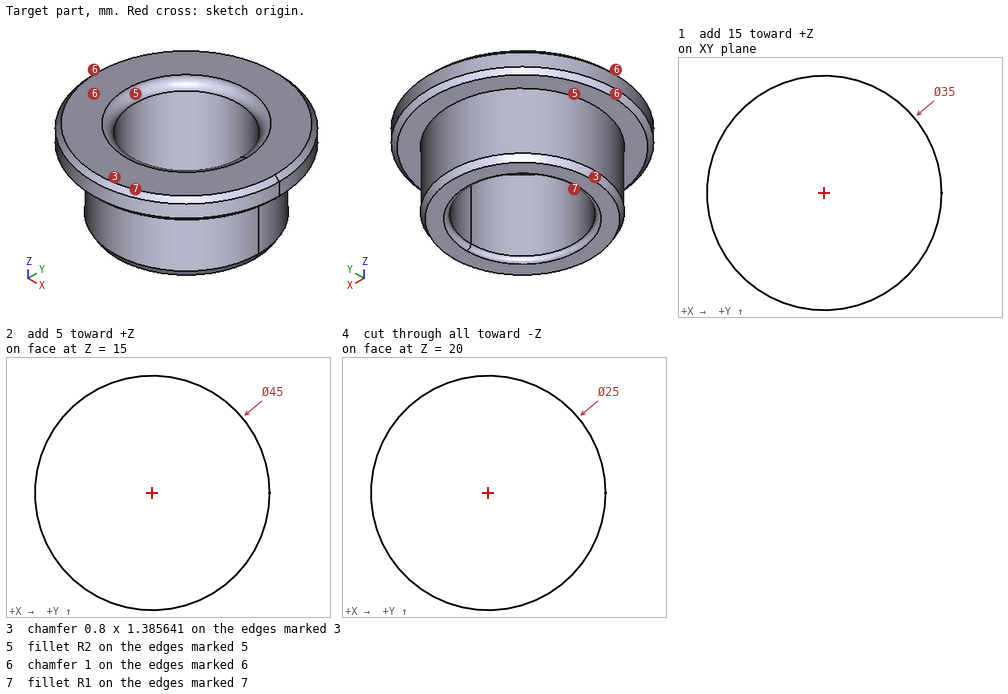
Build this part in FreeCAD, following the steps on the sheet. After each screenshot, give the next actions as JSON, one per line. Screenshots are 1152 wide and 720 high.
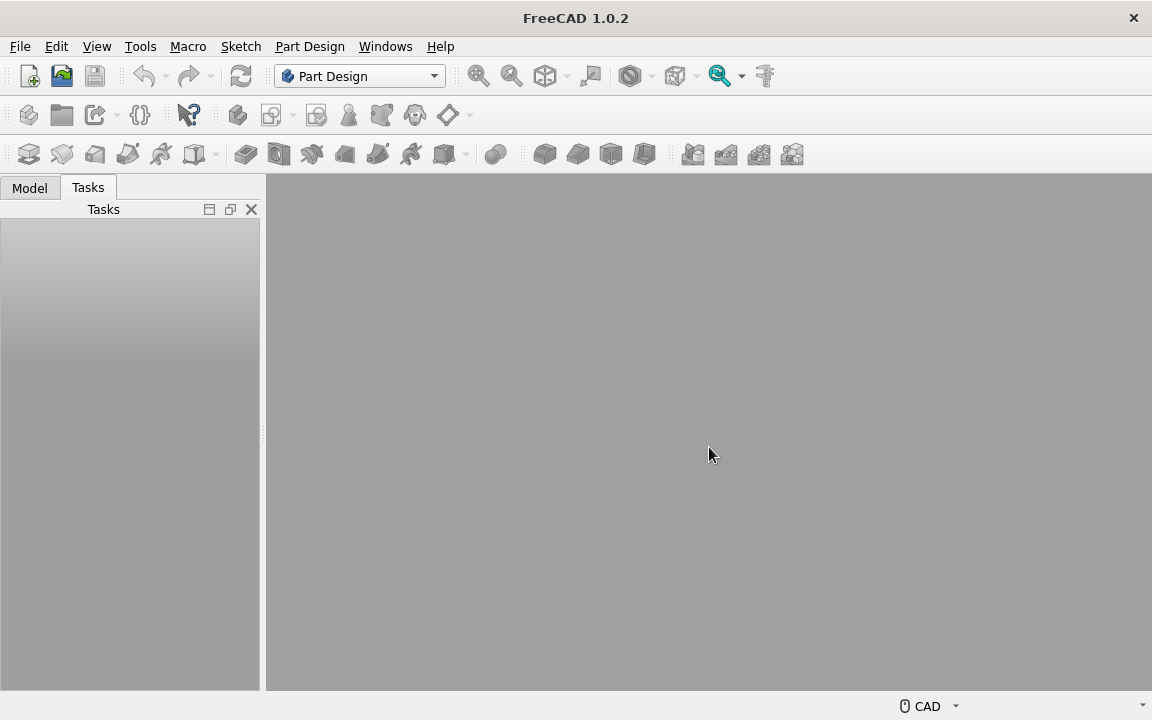
{"action": "left_click", "coordinate": [29, 76]}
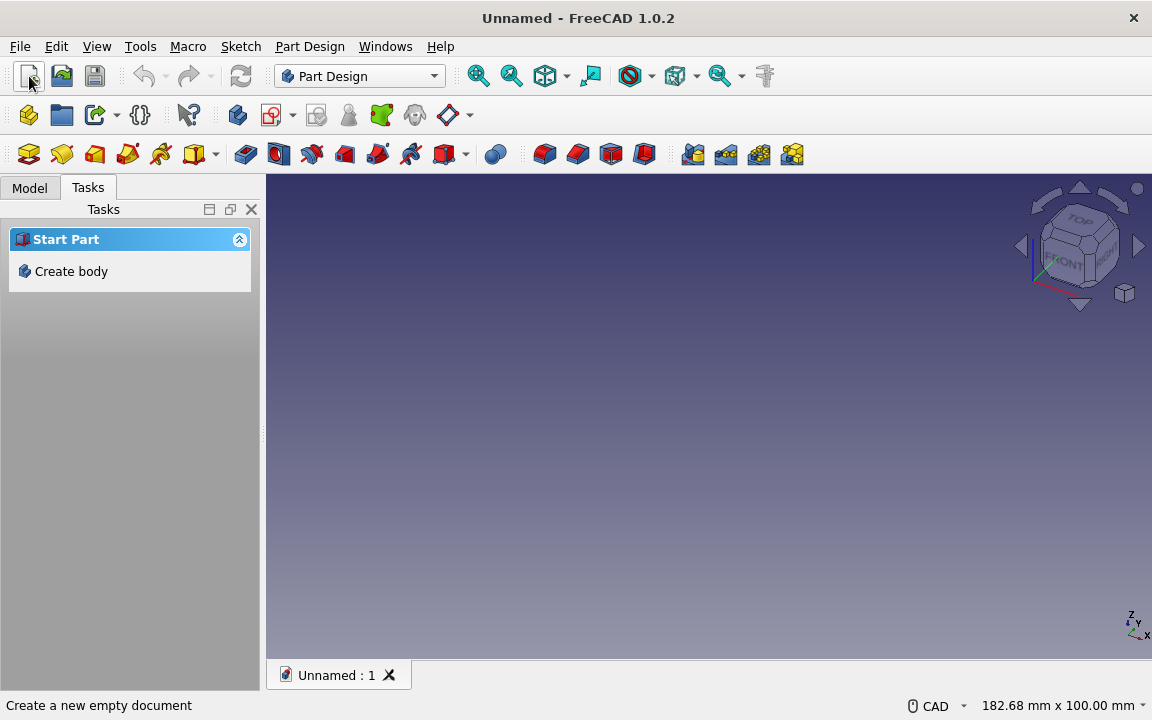
{"action": "left_click", "coordinate": [270, 116]}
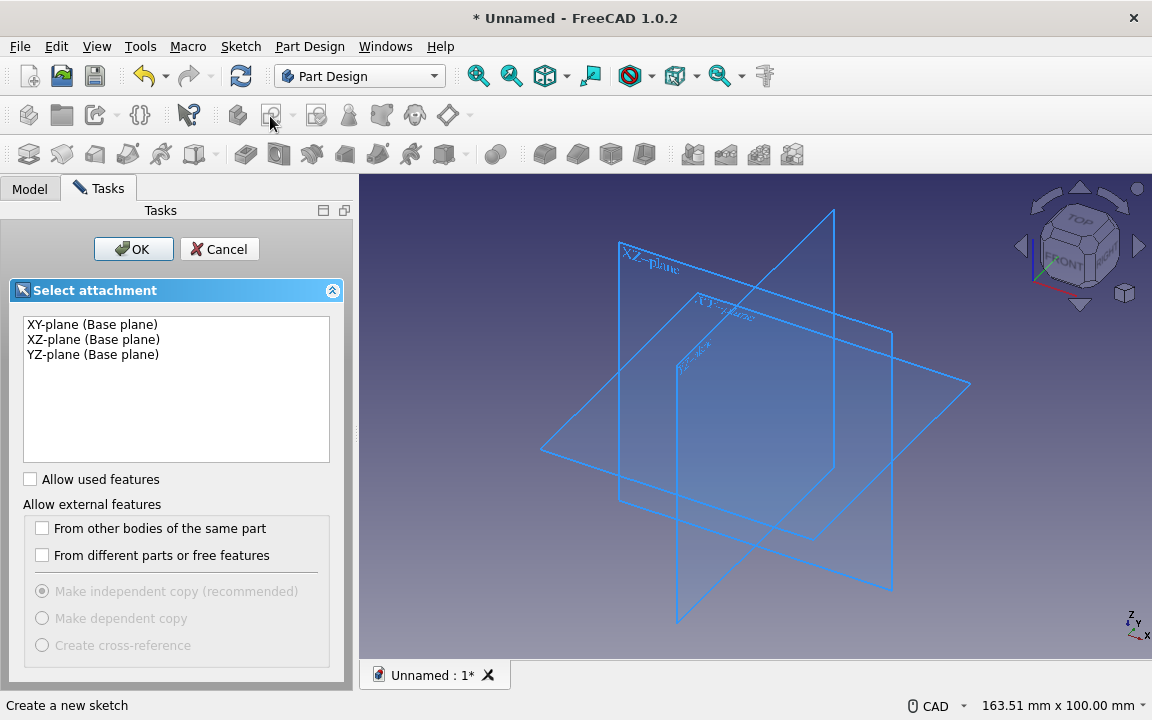
{"action": "left_click", "coordinate": [84, 324]}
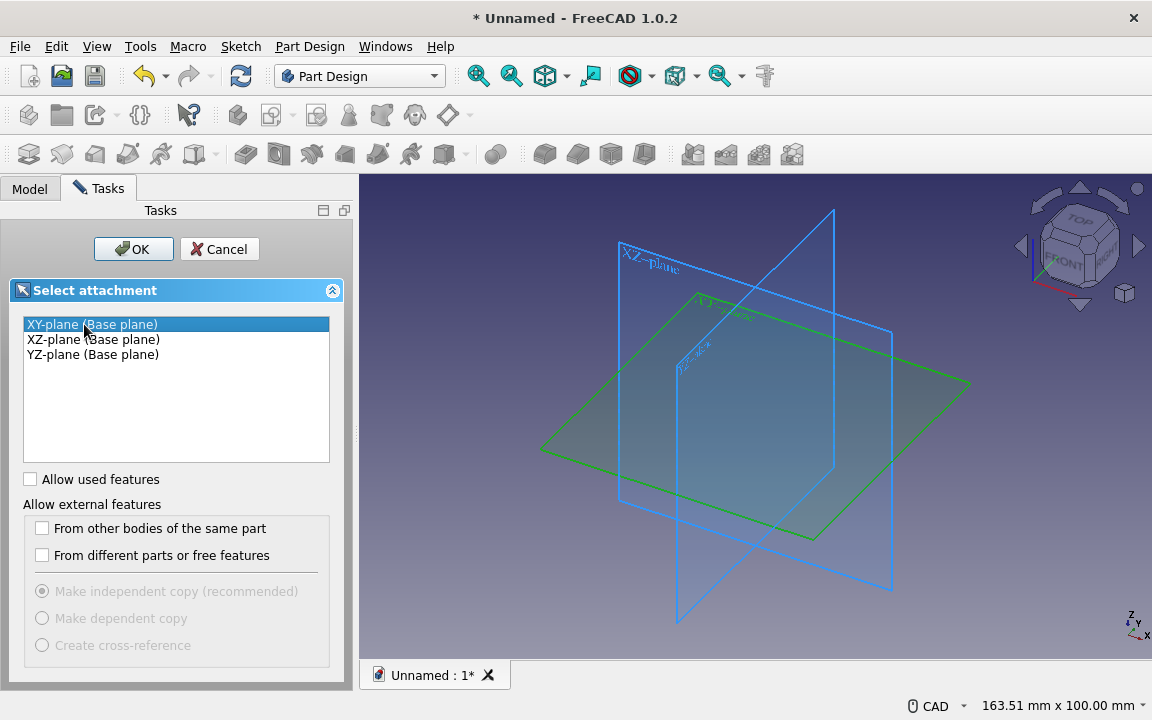
{"action": "left_click", "coordinate": [134, 249]}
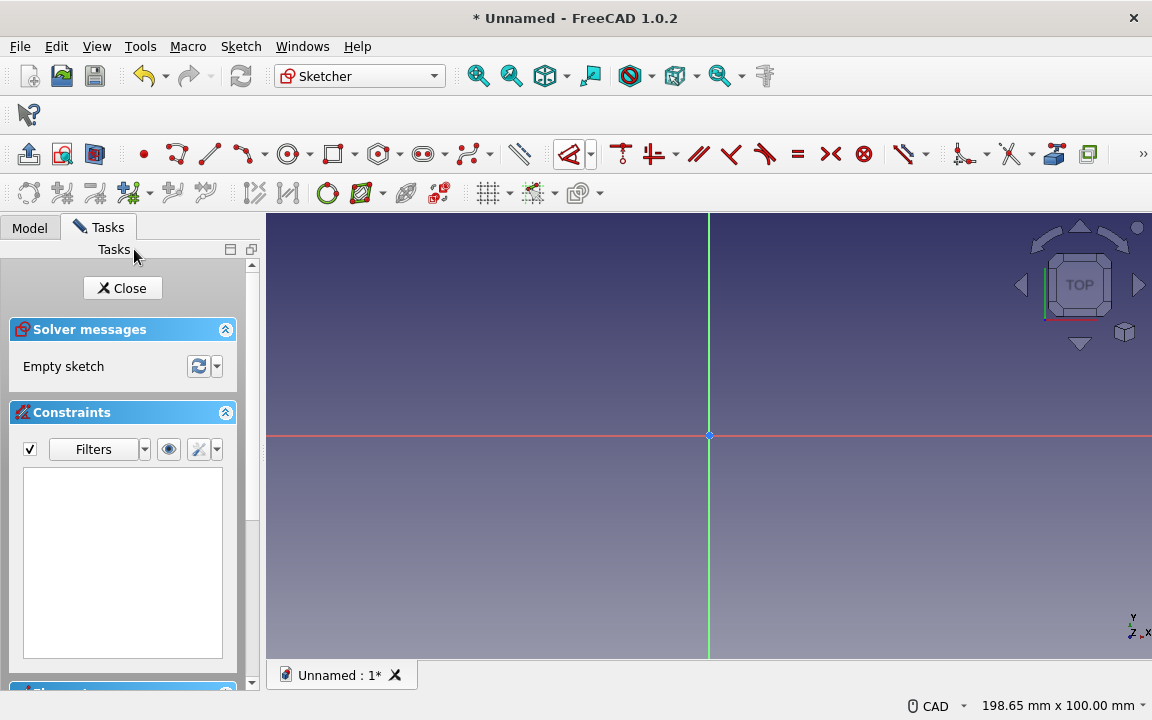
{"action": "scroll", "coordinate": [792, 436], "scroll_direction": "up", "scroll_amount": 3}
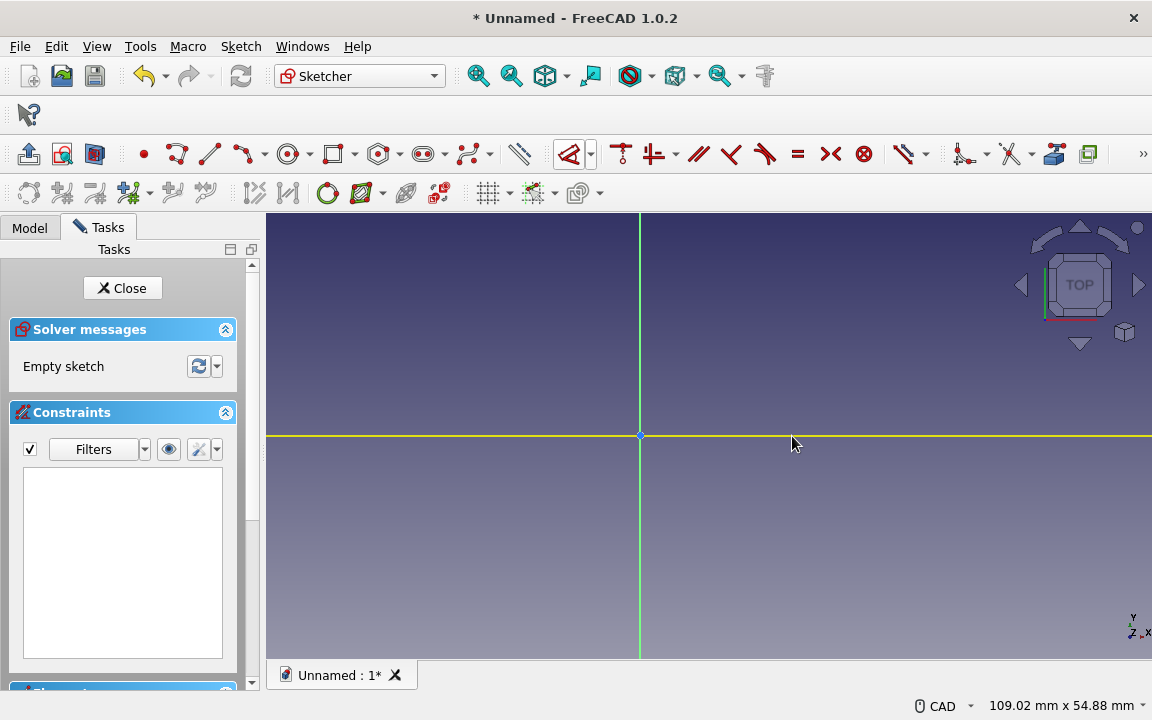
{"action": "key", "text": "g c"}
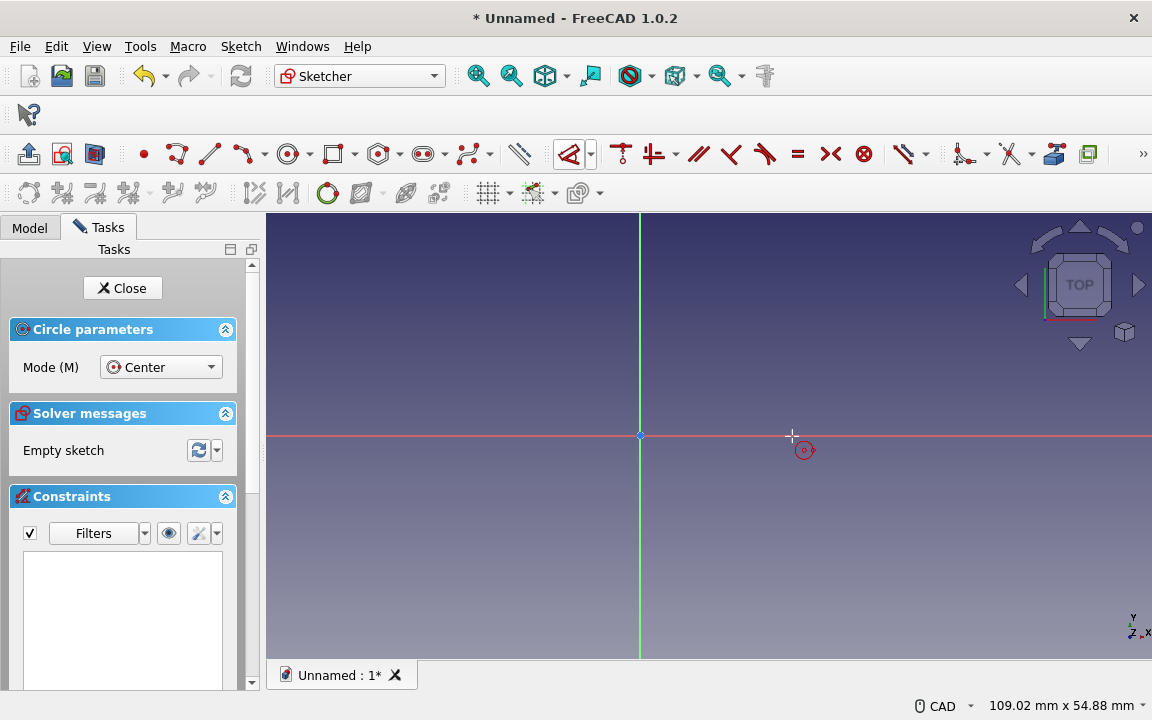
{"action": "left_click", "coordinate": [640, 436]}
{"action": "left_click", "coordinate": [741, 335]}
{"action": "key", "text": "Escape"}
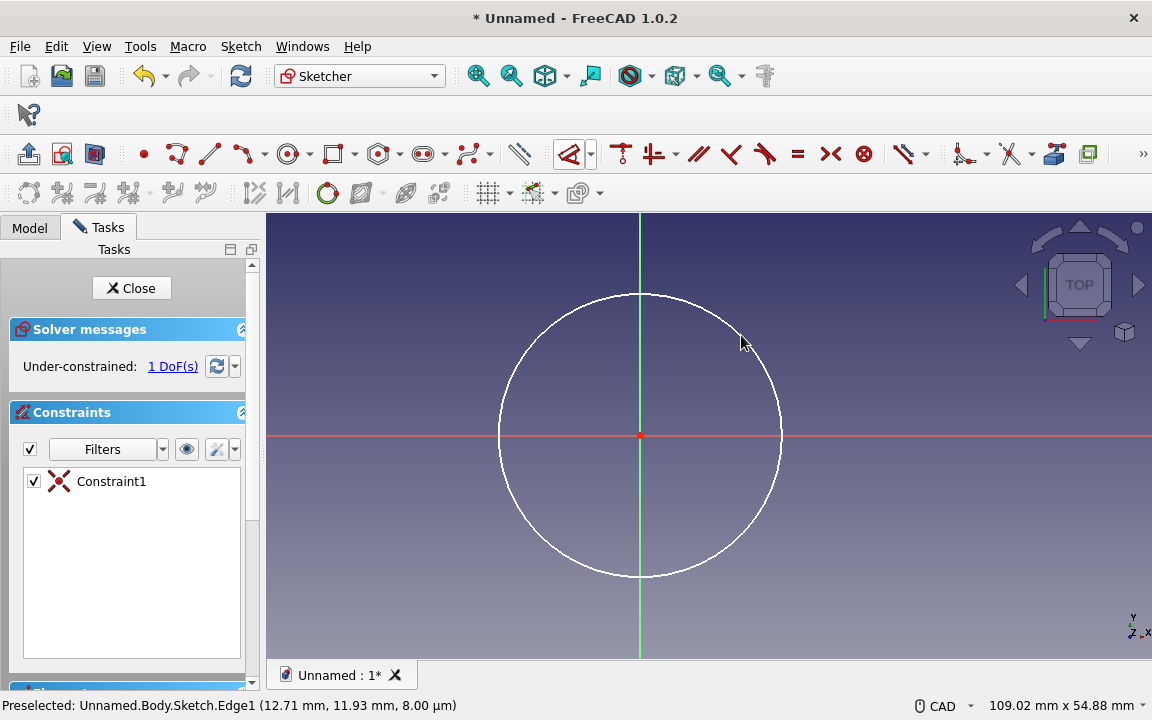
{"action": "left_click", "coordinate": [568, 154]}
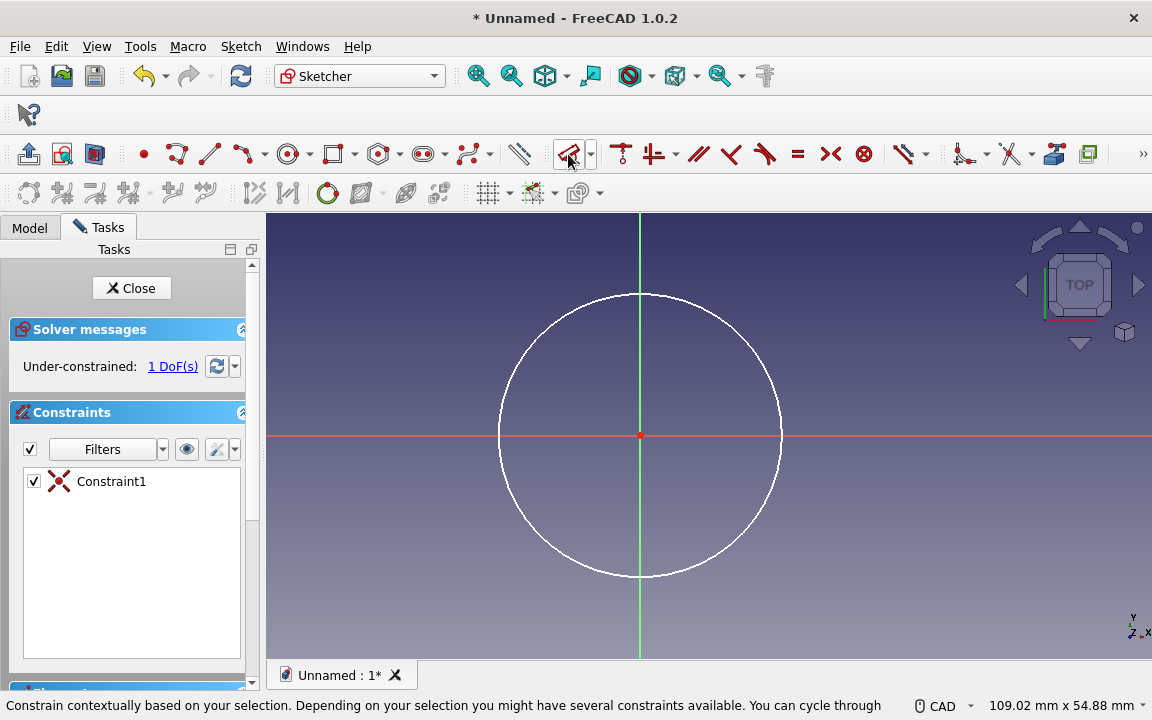
{"action": "left_click", "coordinate": [740, 335]}
{"action": "left_click", "coordinate": [763, 312]}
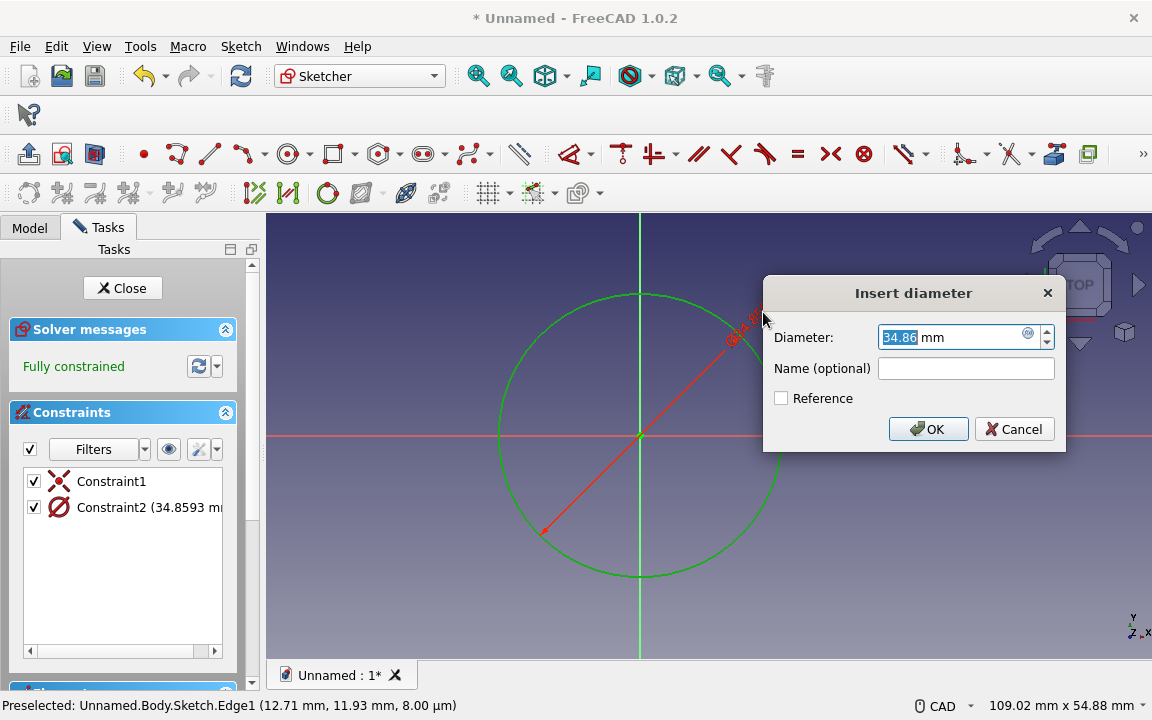
{"action": "type", "text": "35"}
{"action": "key", "text": "Return"}
{"action": "key", "text": "Escape"}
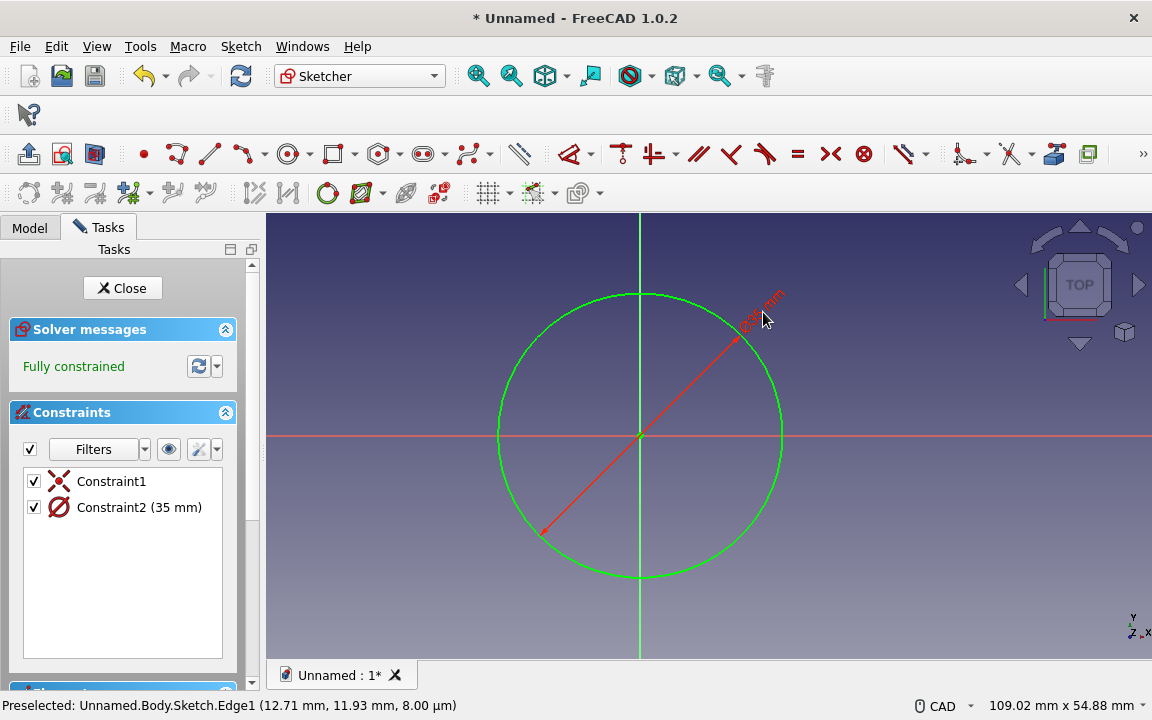
{"action": "left_click", "coordinate": [123, 288]}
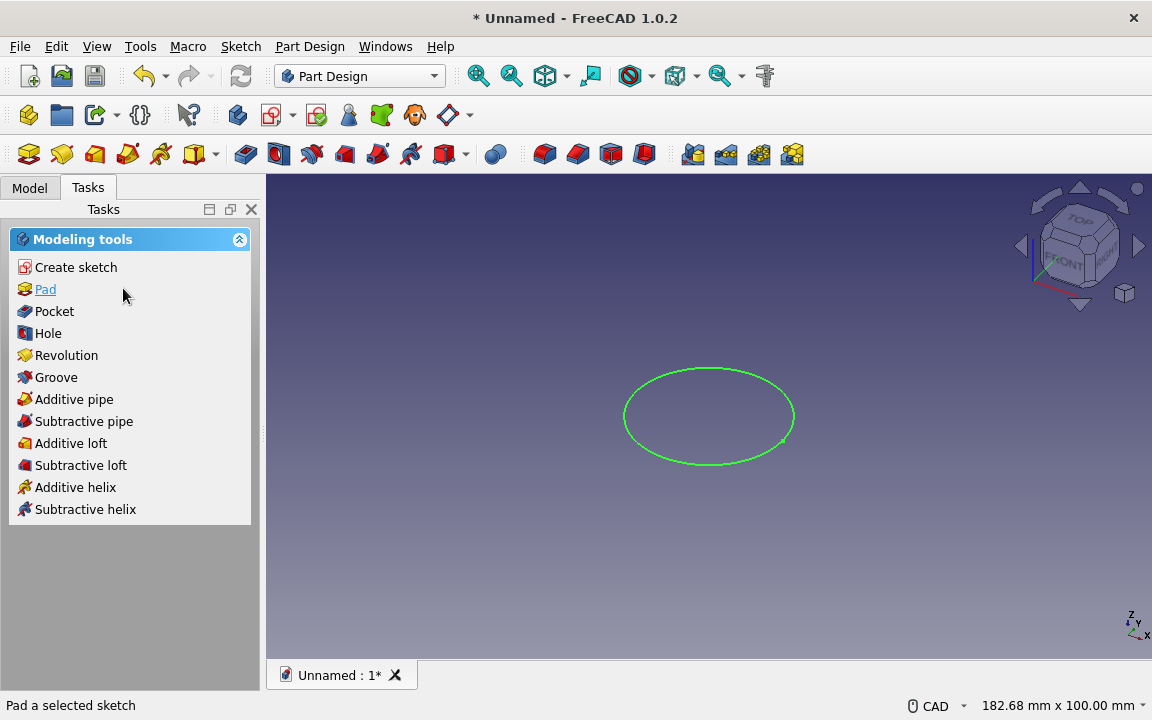
{"action": "left_click", "coordinate": [29, 154]}